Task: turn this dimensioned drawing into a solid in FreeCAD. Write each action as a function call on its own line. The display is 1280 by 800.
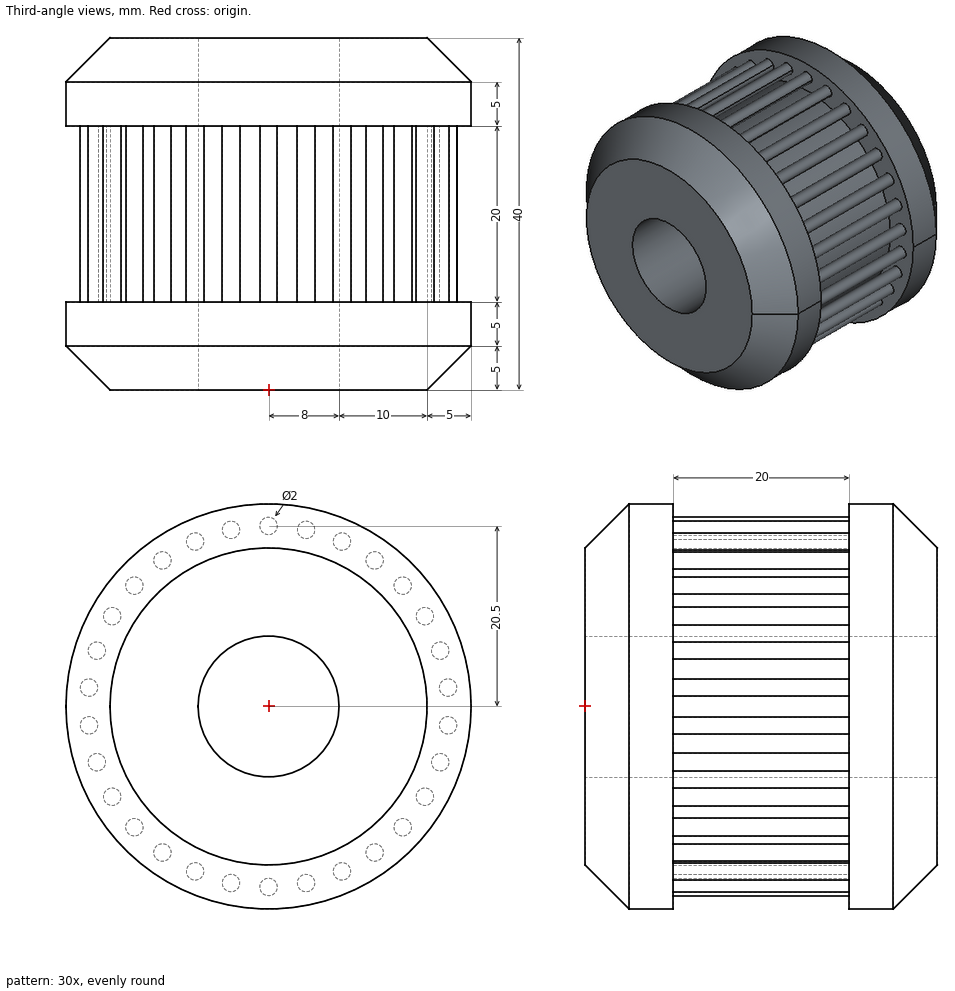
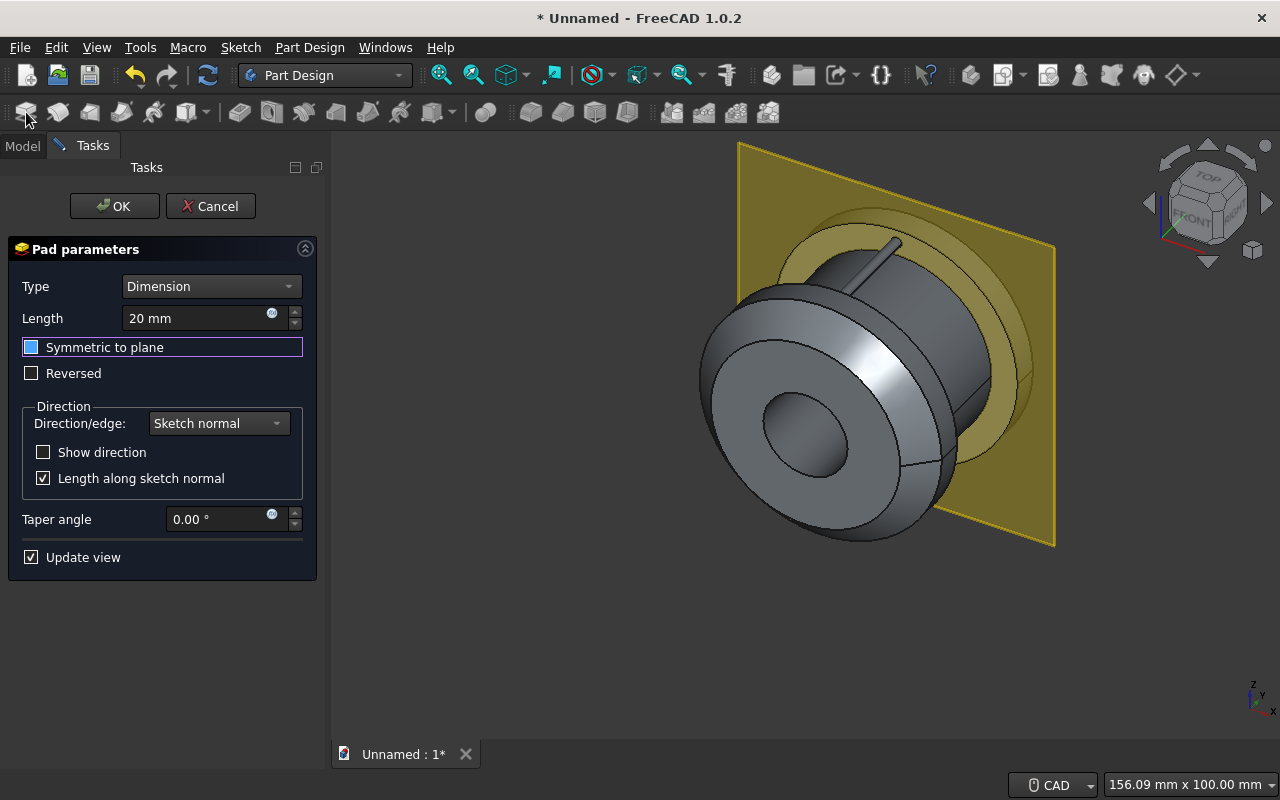
click(115, 206)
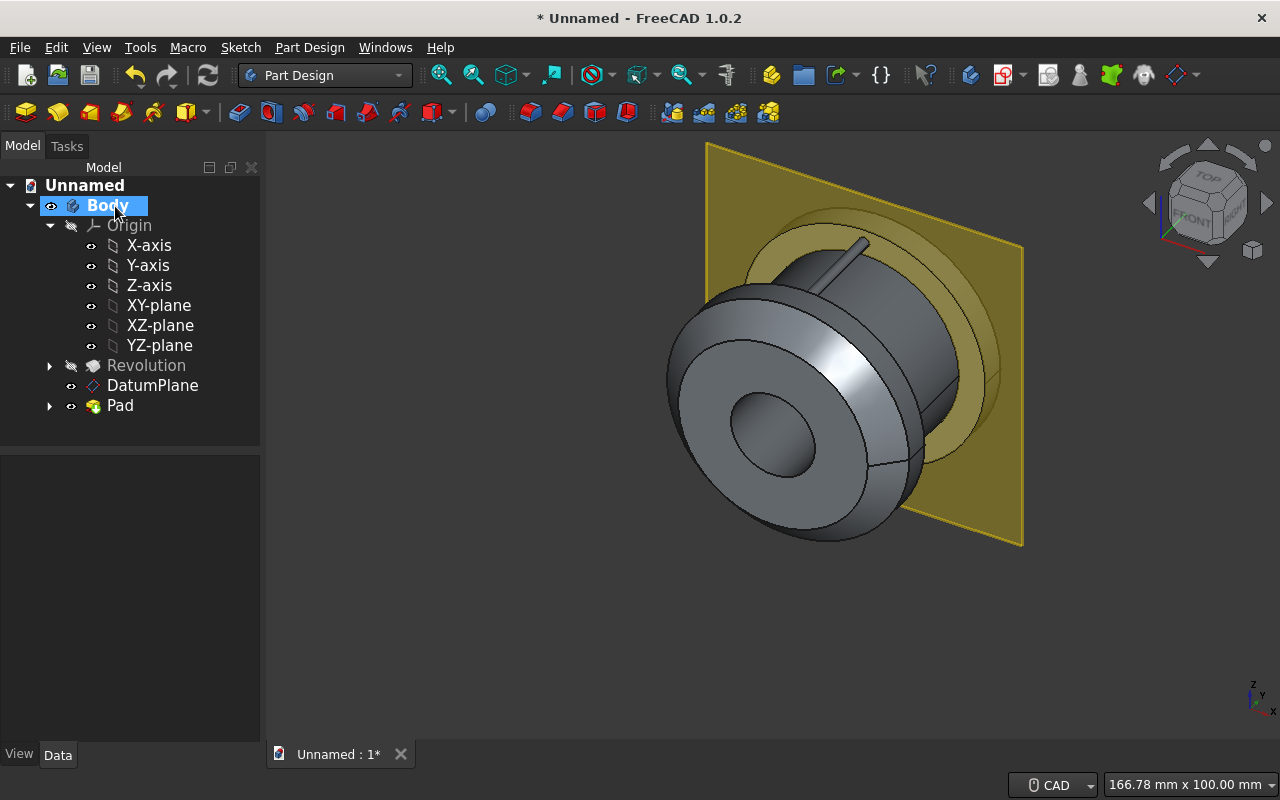
click(116, 386)
key(space)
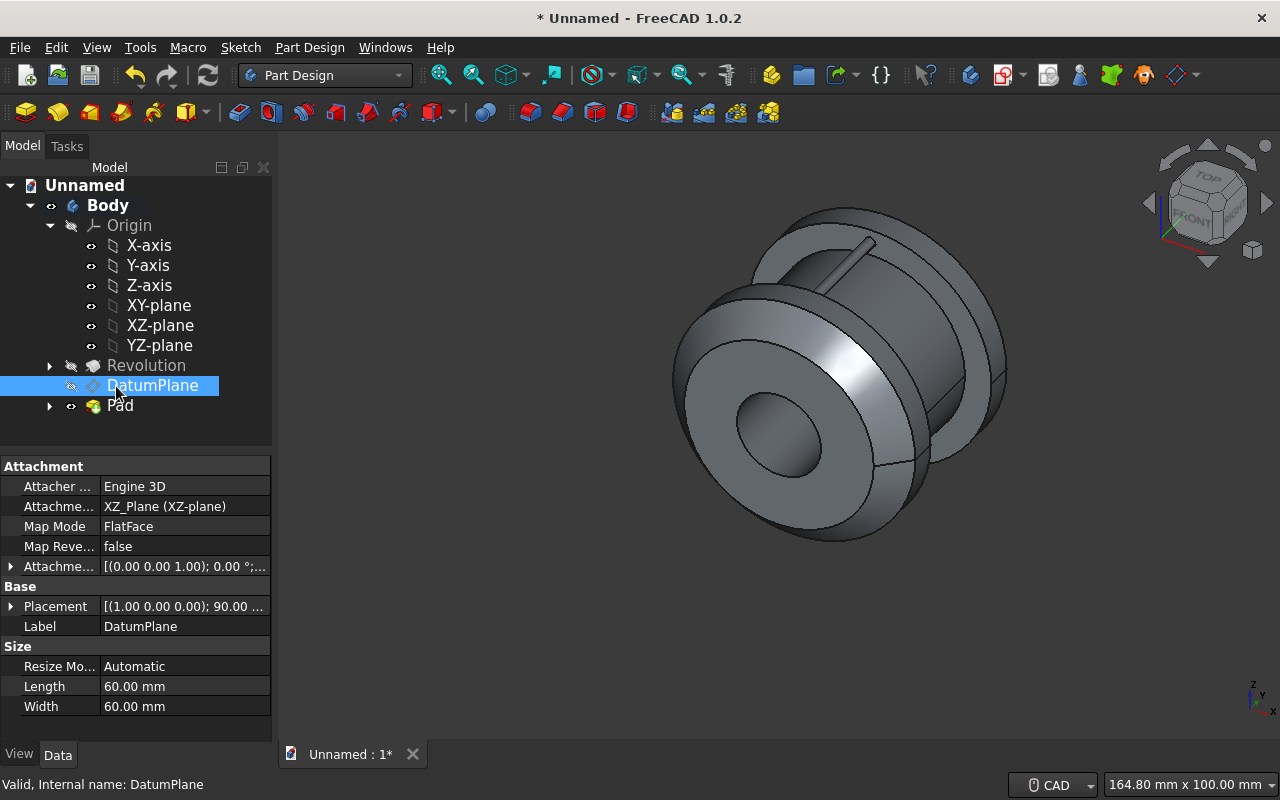
click(116, 406)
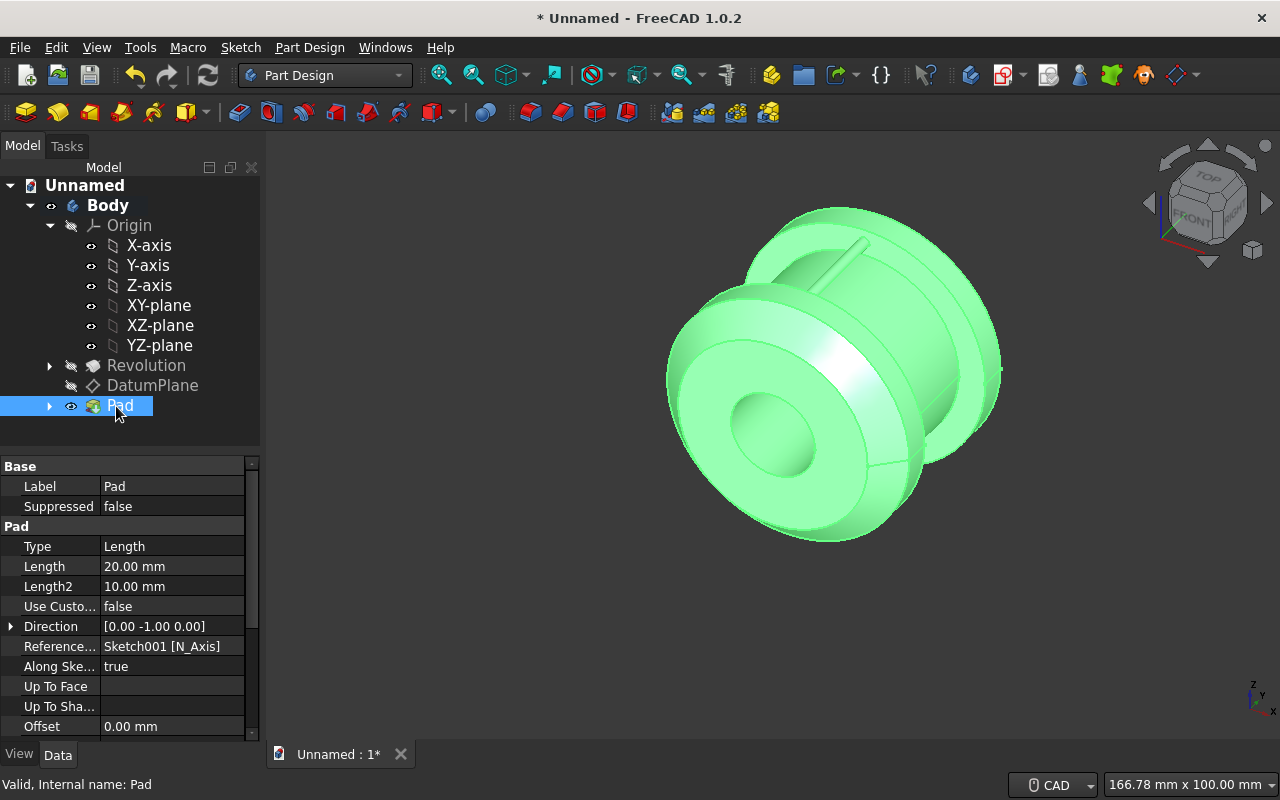
click(736, 112)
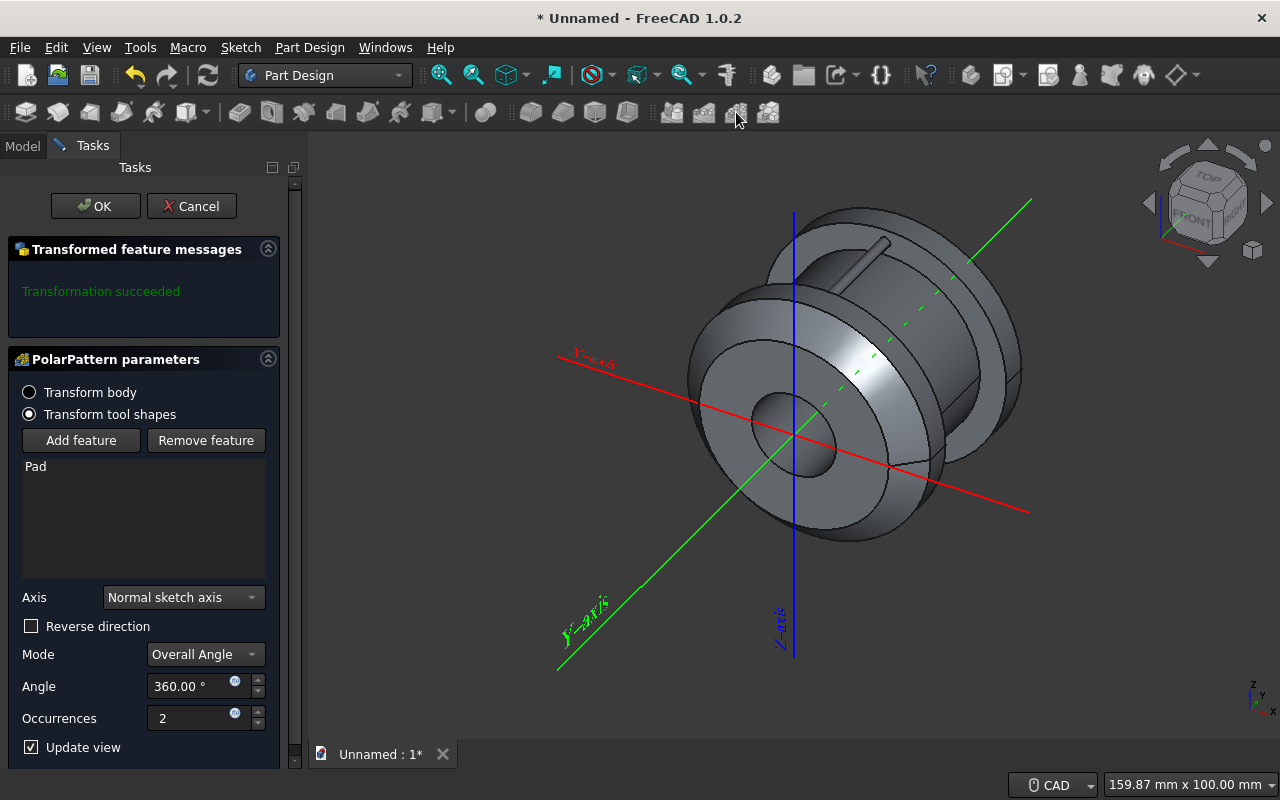
click(184, 598)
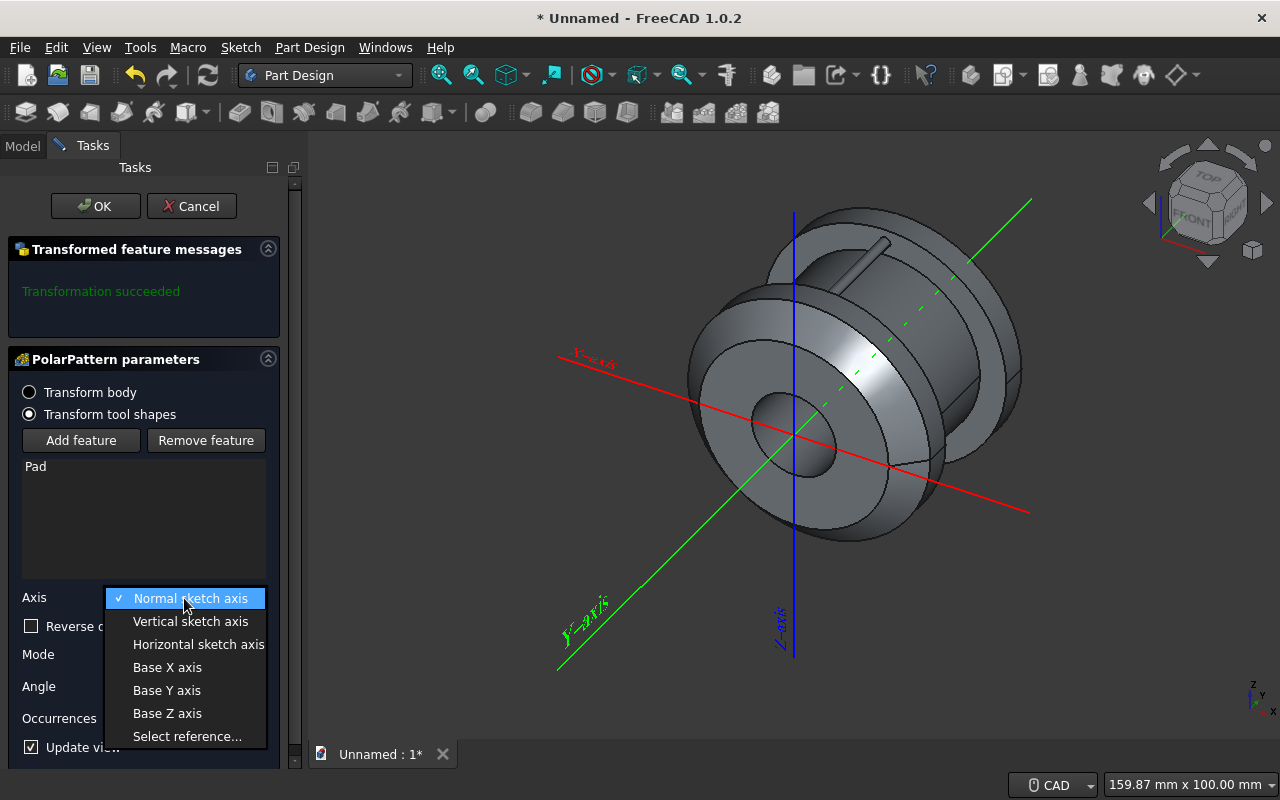
click(184, 690)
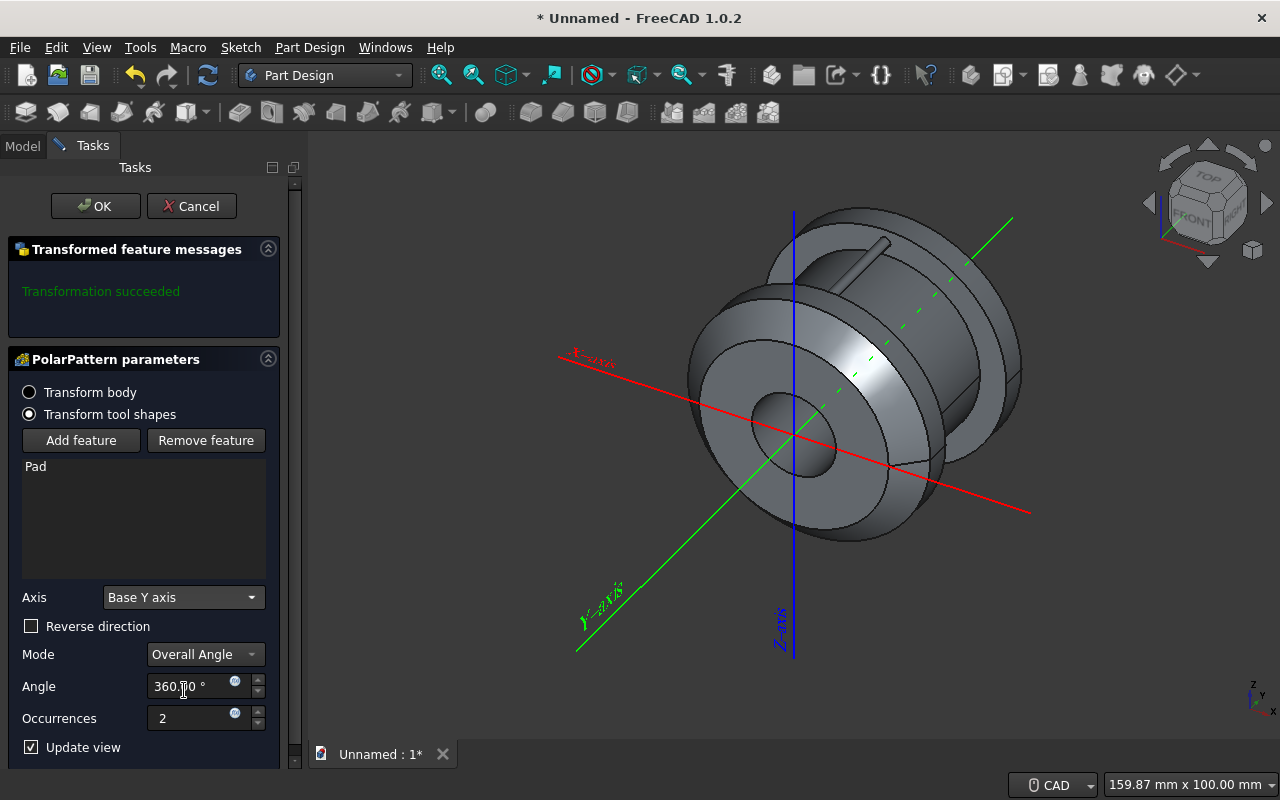
triple_click(198, 718)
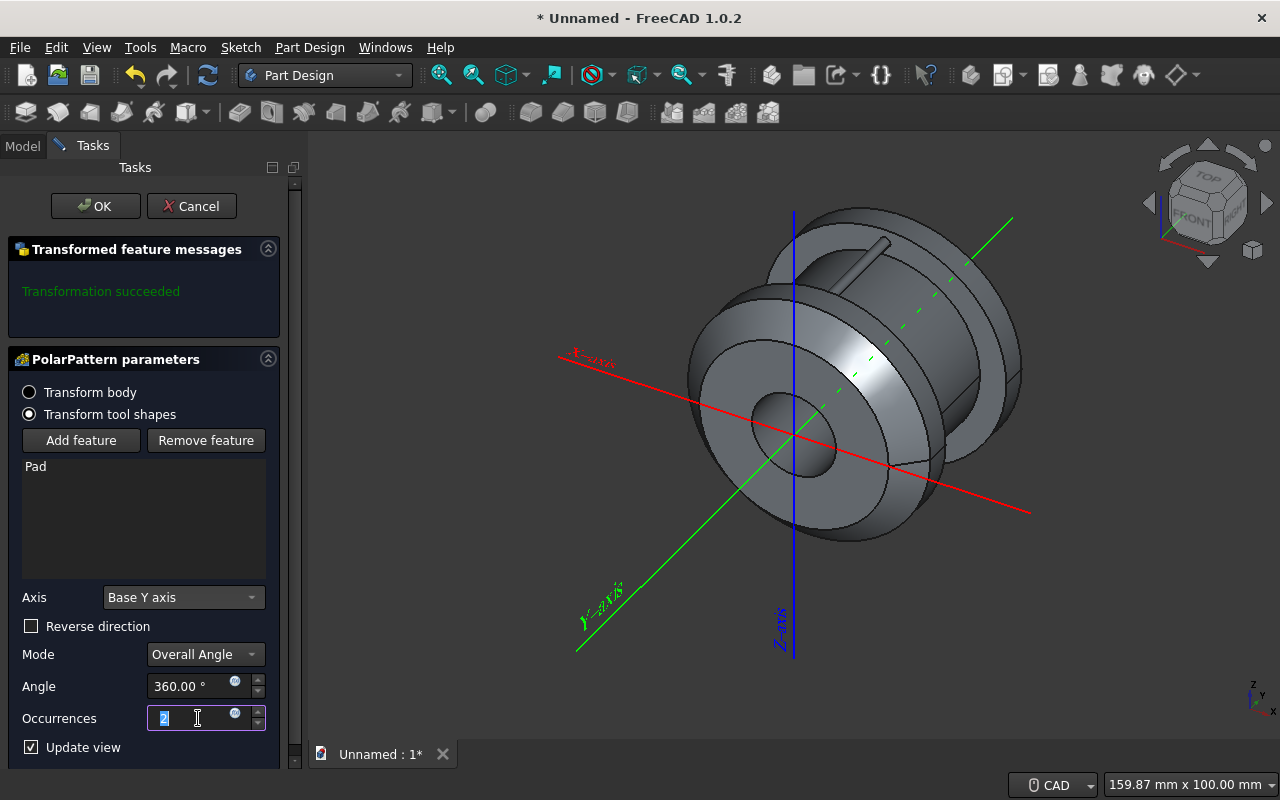
text(30)
key(Tab)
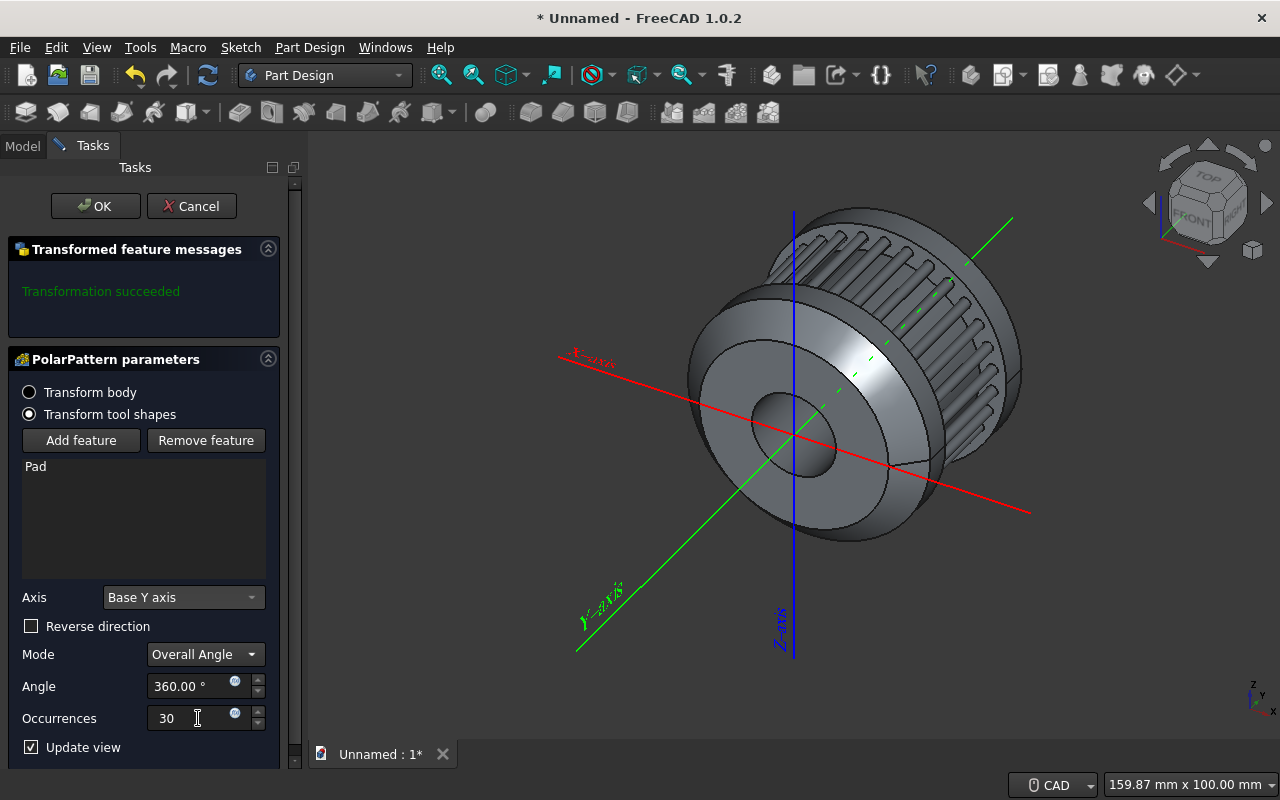
click(96, 206)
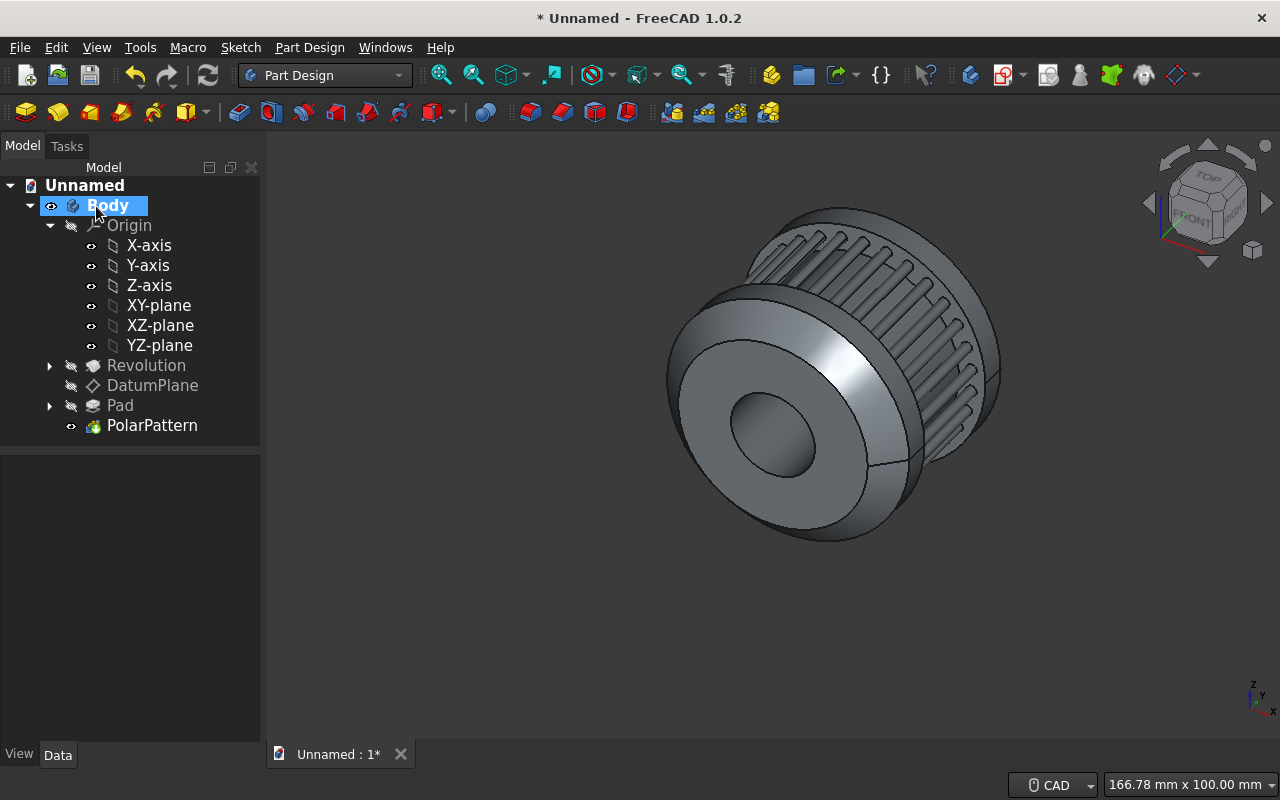
key(0)